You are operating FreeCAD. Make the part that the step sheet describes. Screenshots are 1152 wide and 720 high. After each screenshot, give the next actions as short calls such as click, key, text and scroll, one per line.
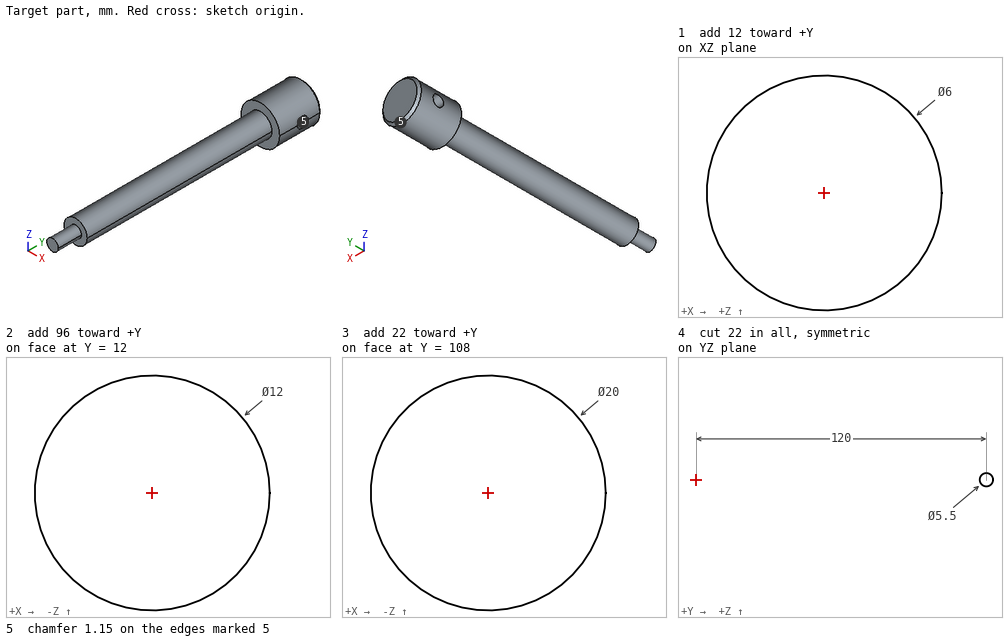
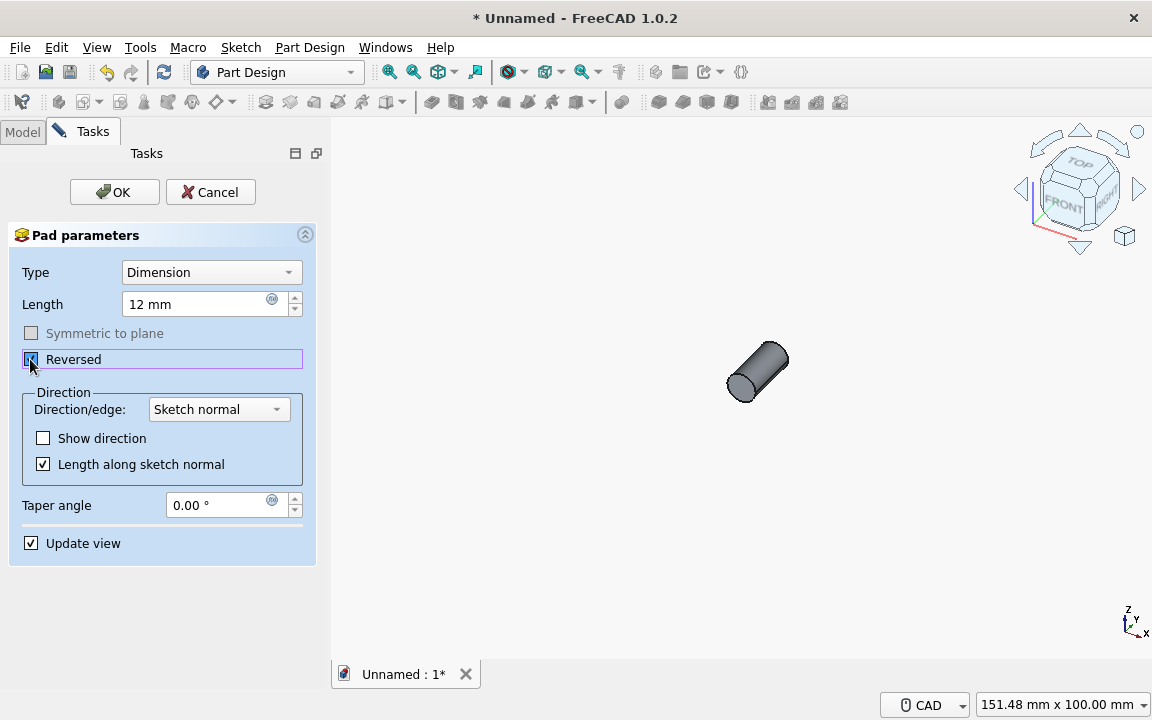
click(115, 192)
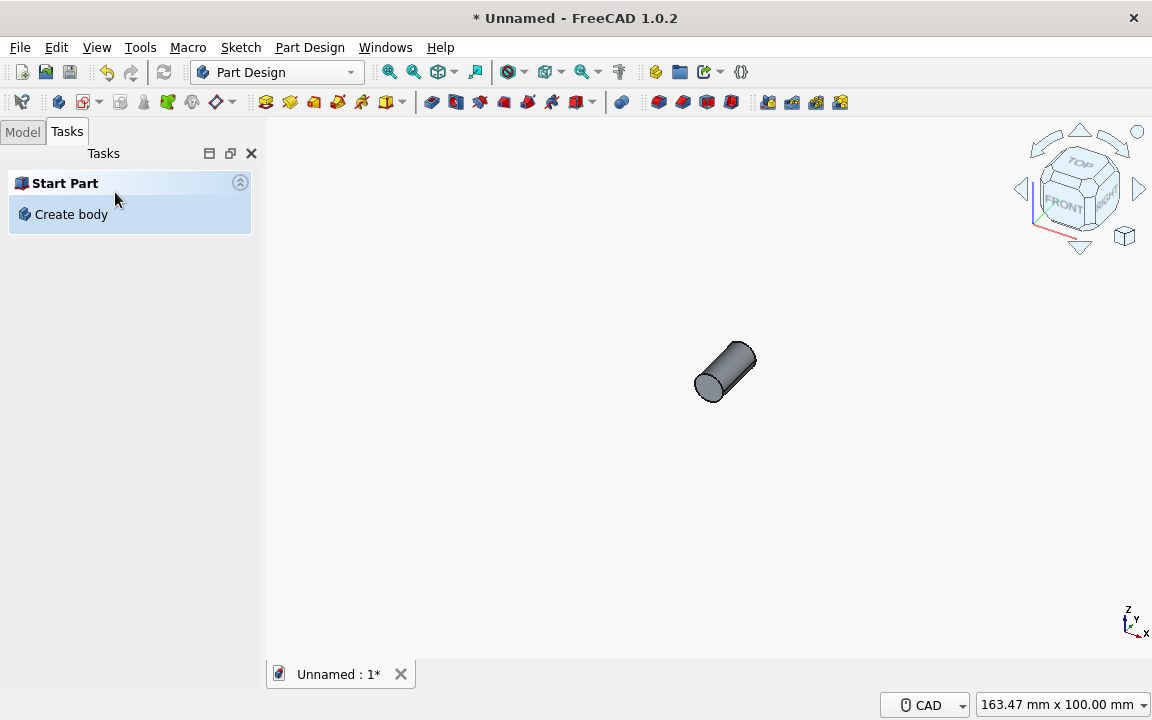
click(390, 72)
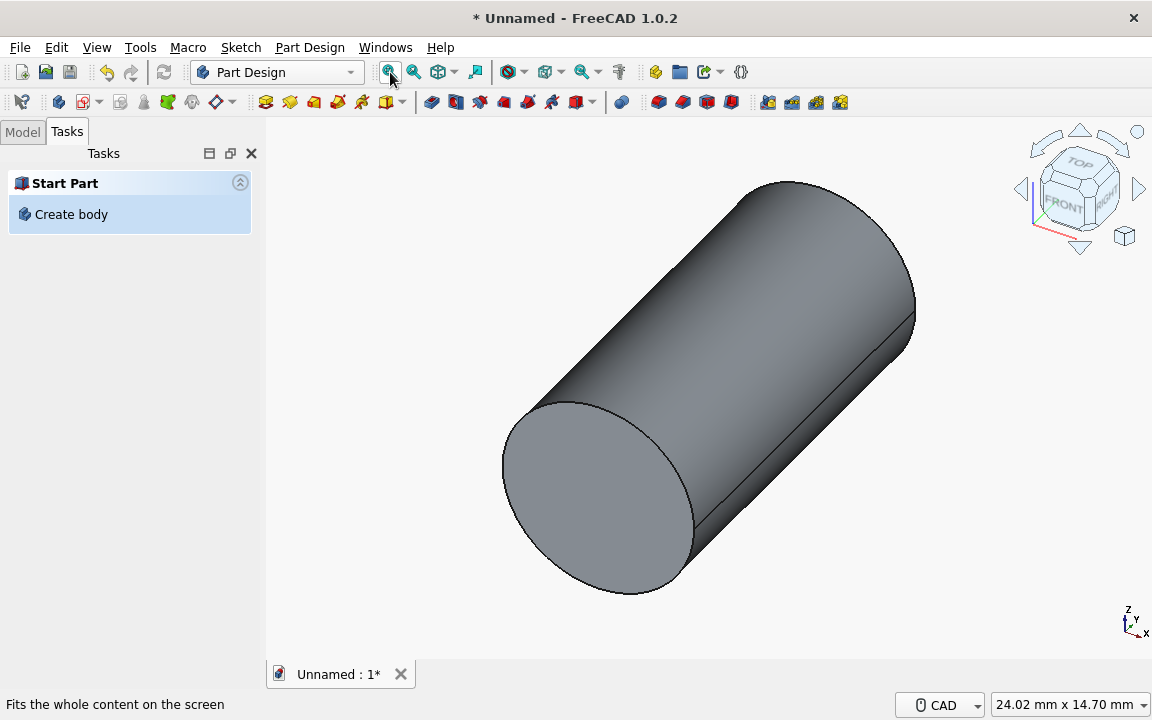
key(4)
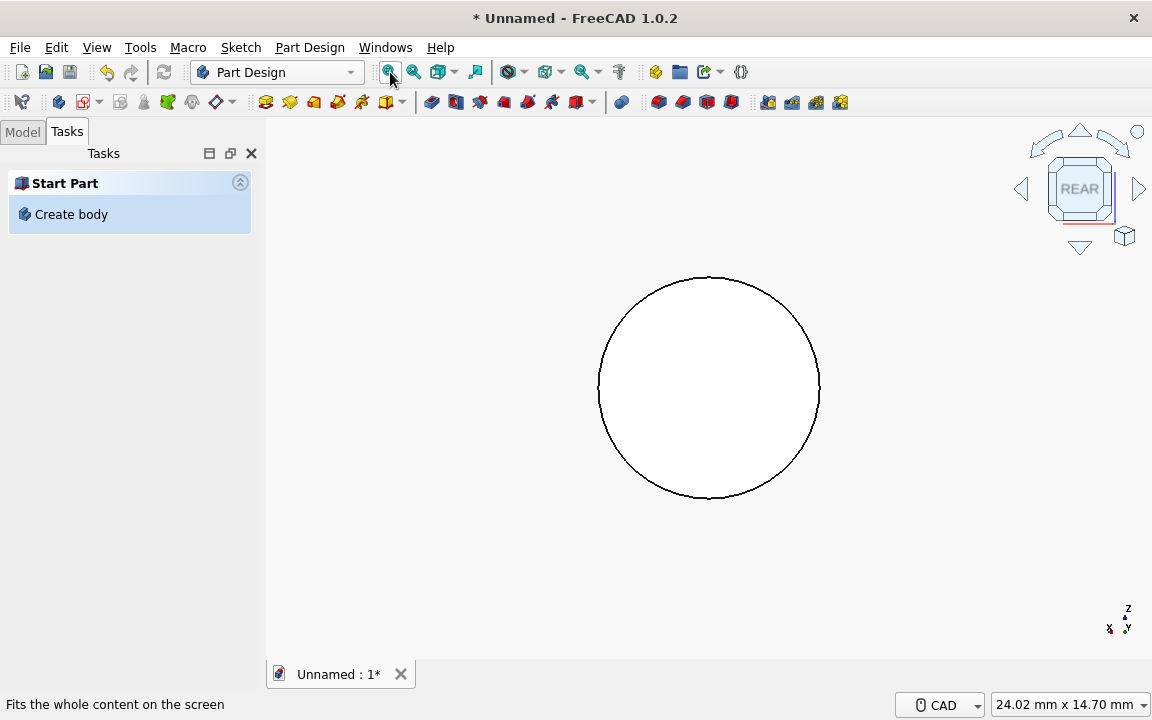
click(390, 72)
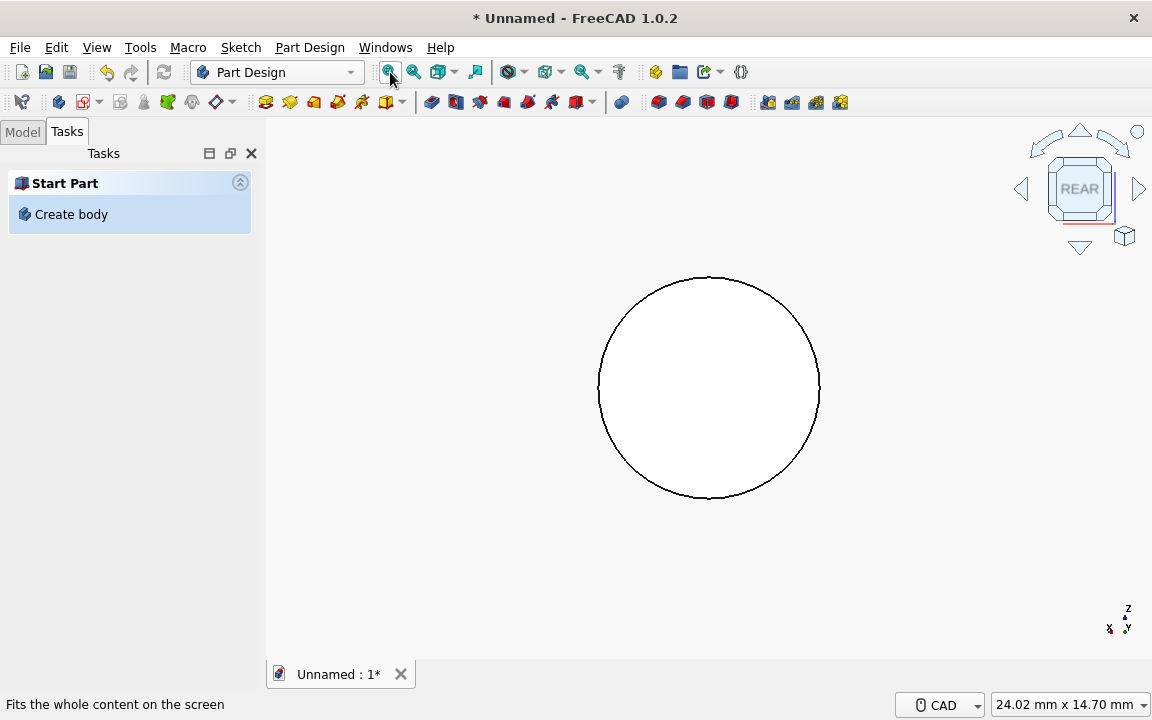
click(709, 387)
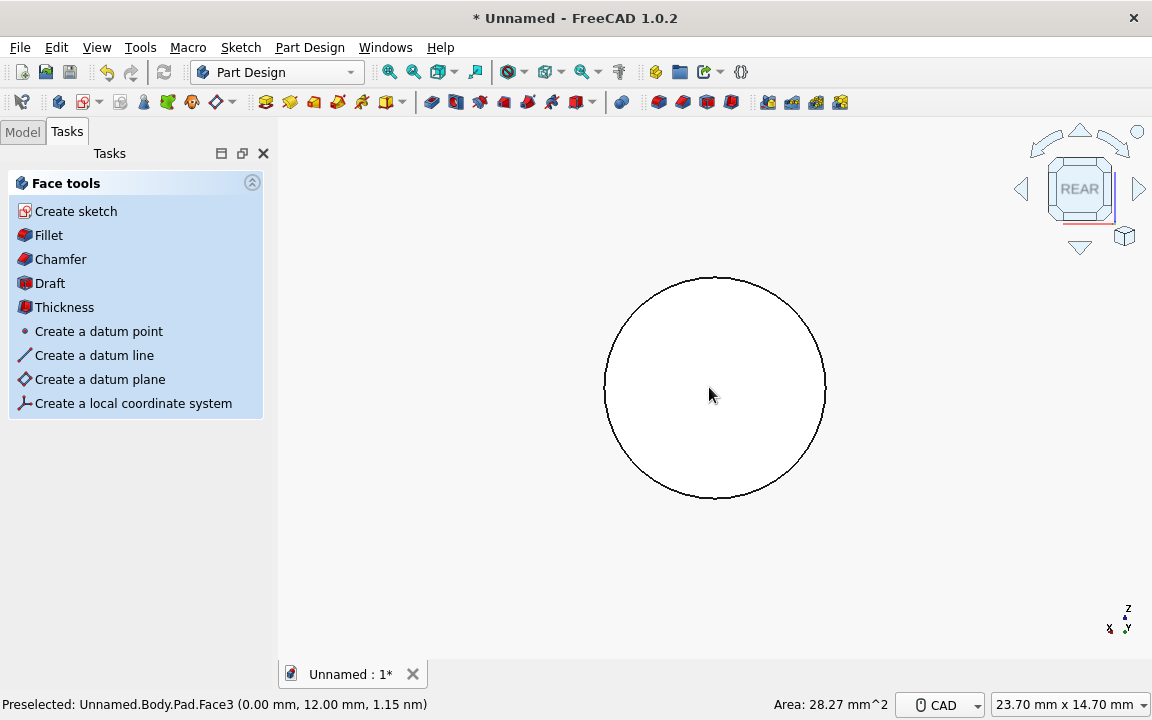
click(84, 102)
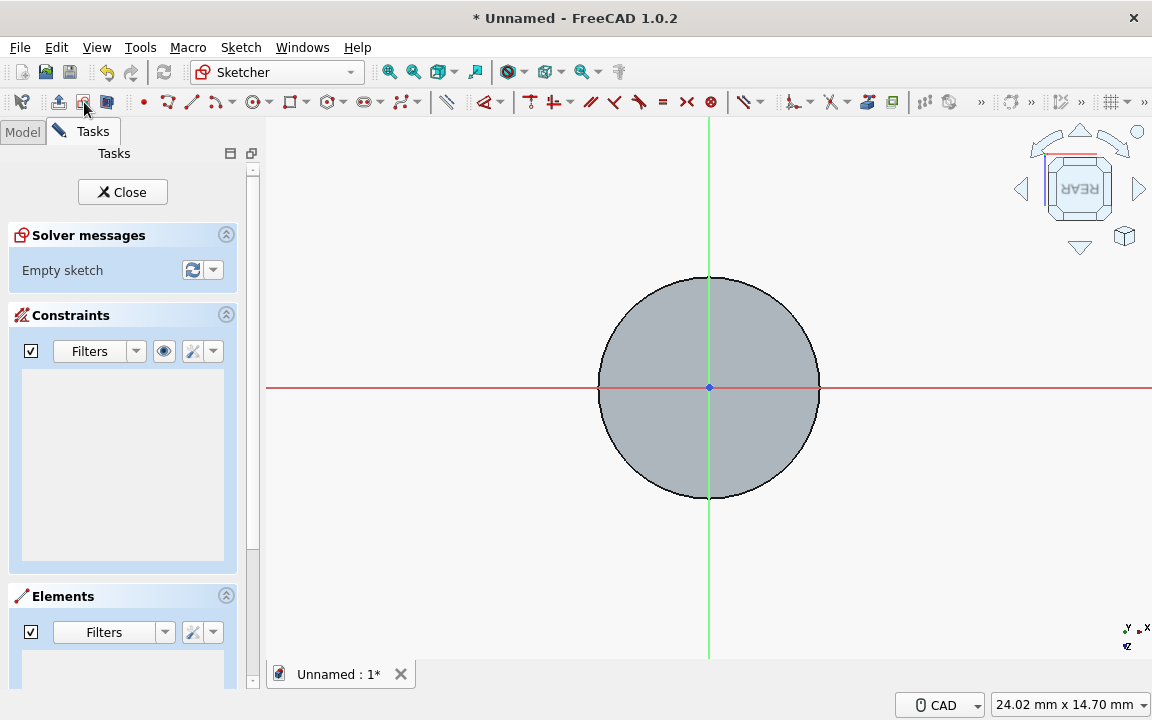
scroll(331, 388, down, 1)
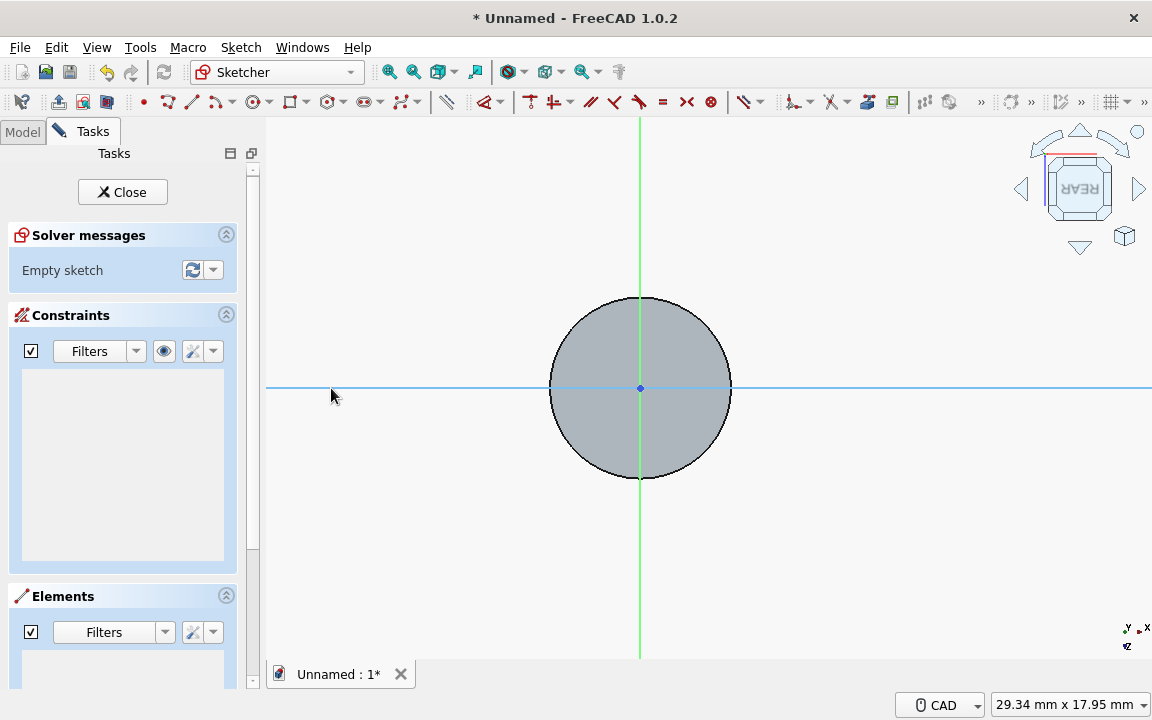
click(254, 102)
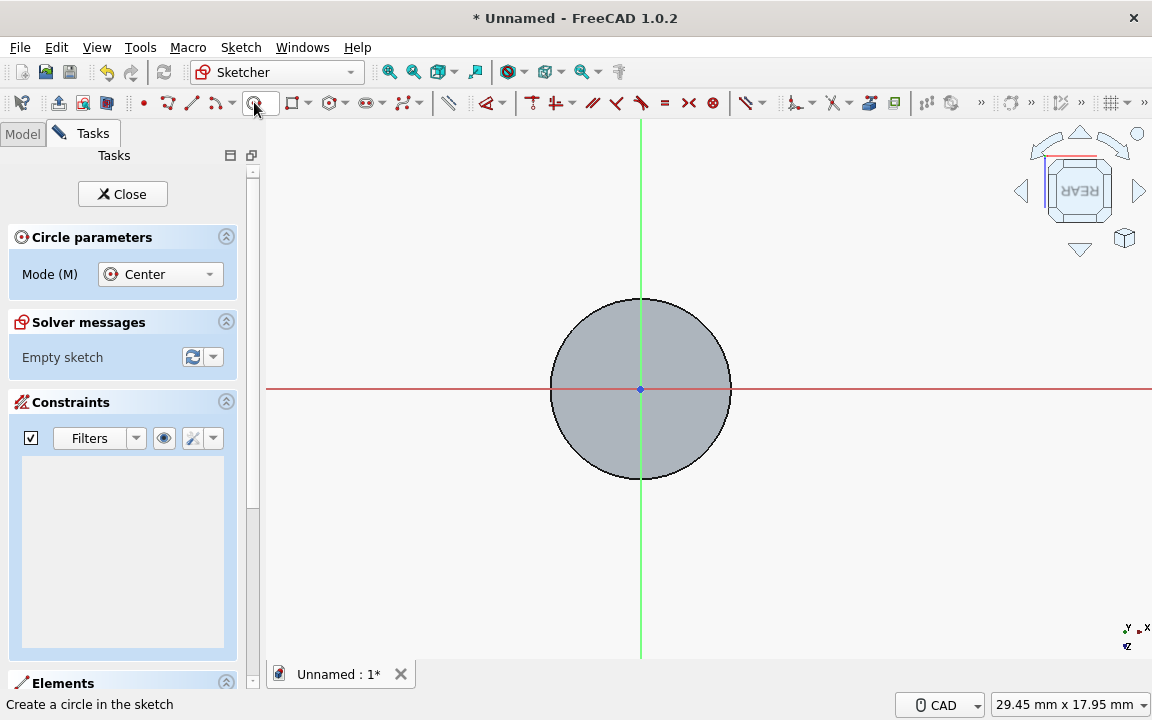
click(641, 389)
move(768, 261)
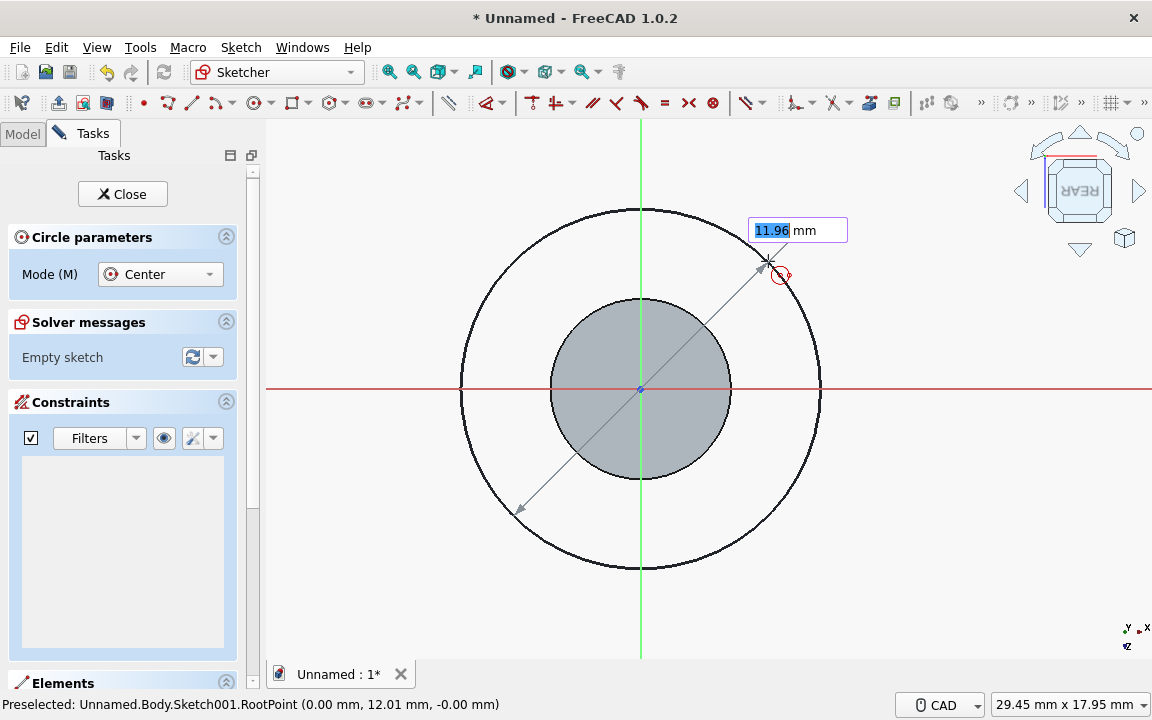
text(12)
key(Return)
key(Escape)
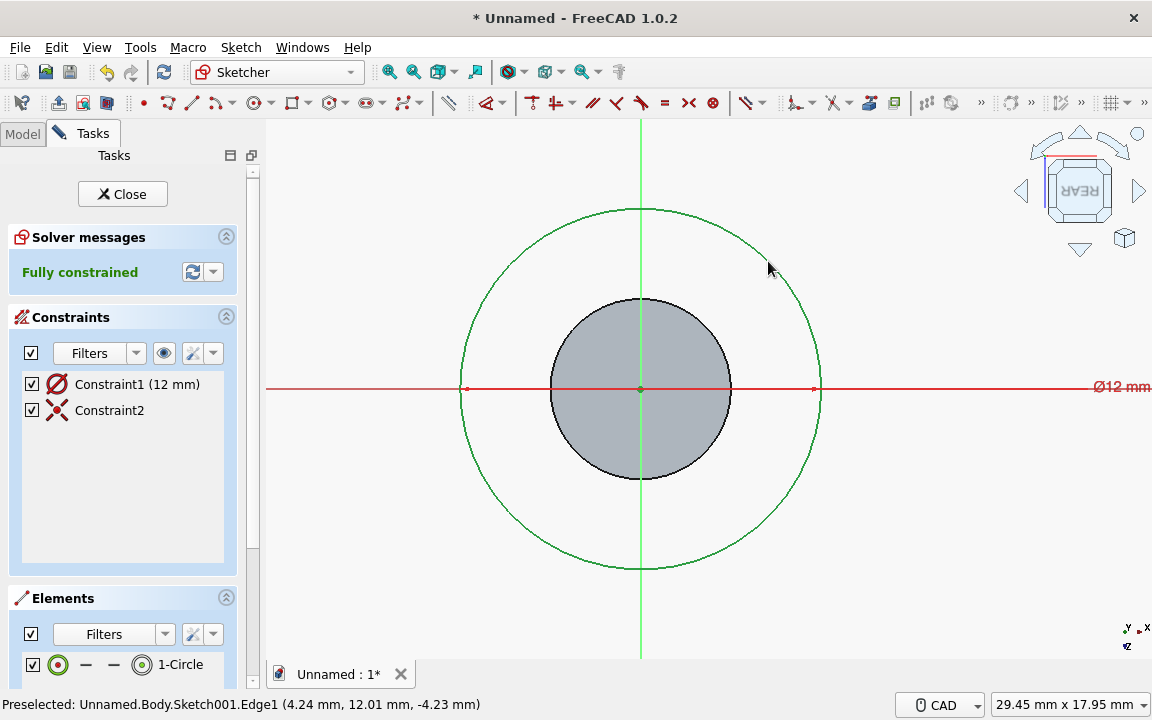
click(123, 194)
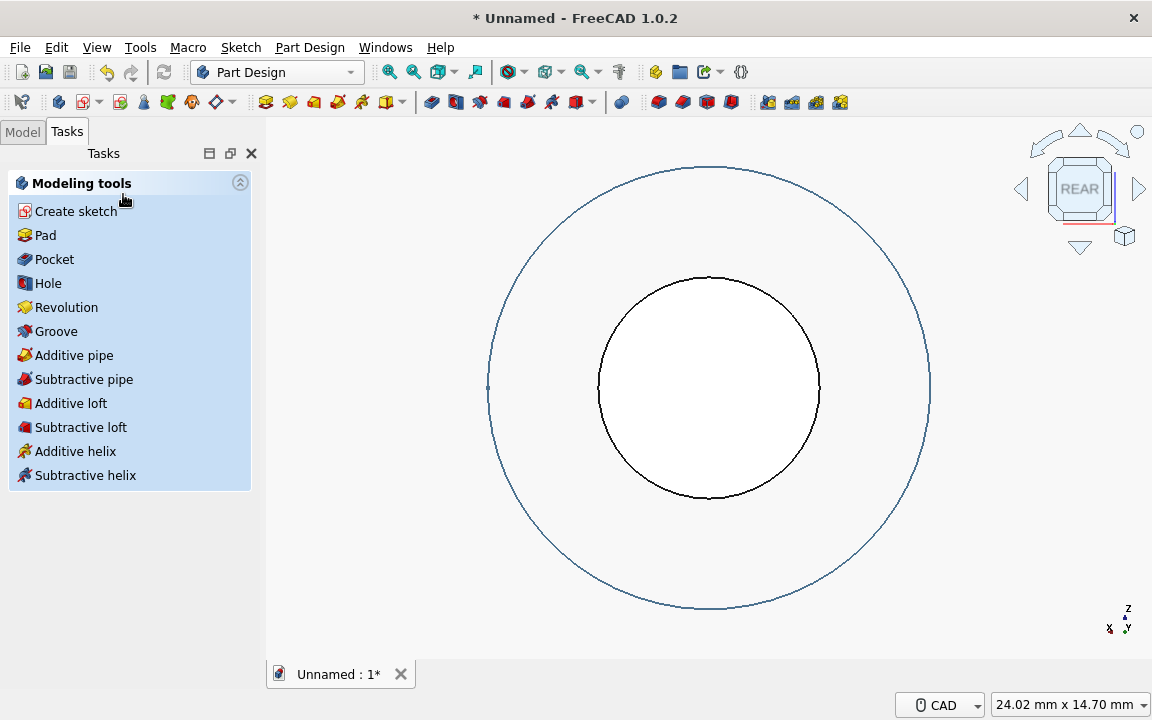
click(266, 102)